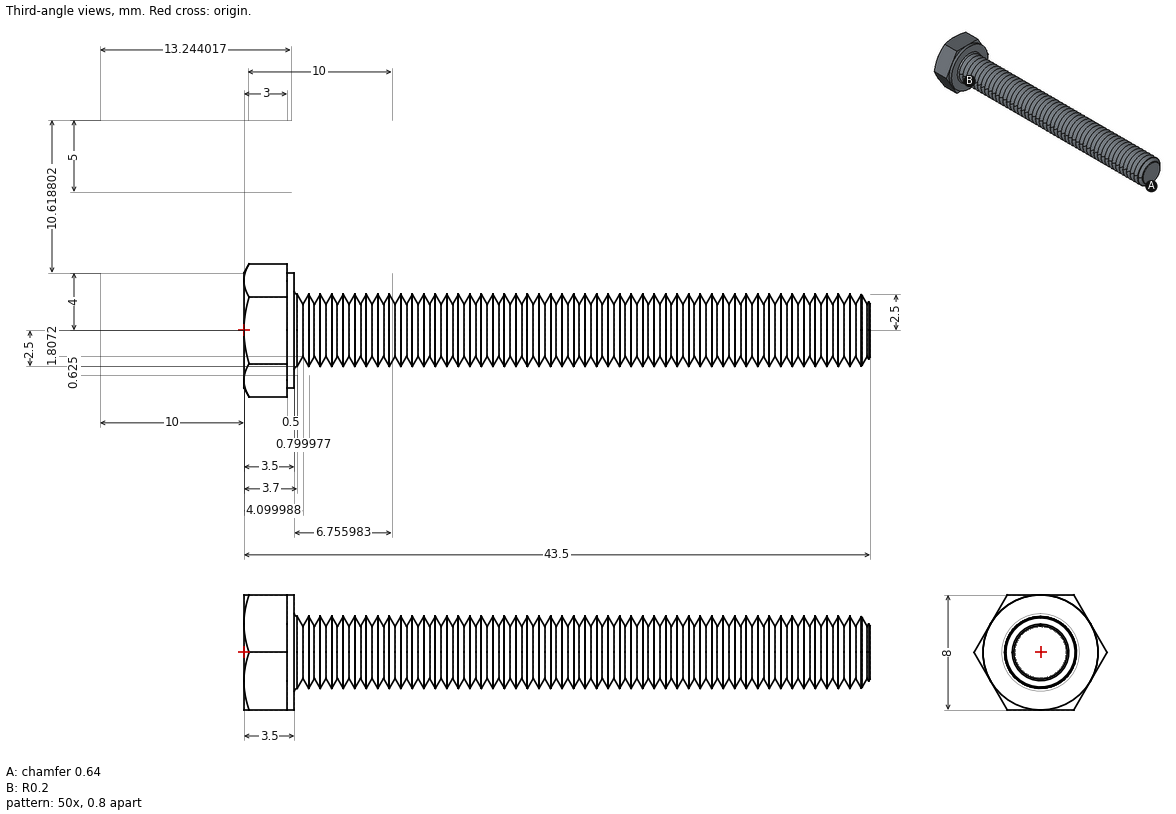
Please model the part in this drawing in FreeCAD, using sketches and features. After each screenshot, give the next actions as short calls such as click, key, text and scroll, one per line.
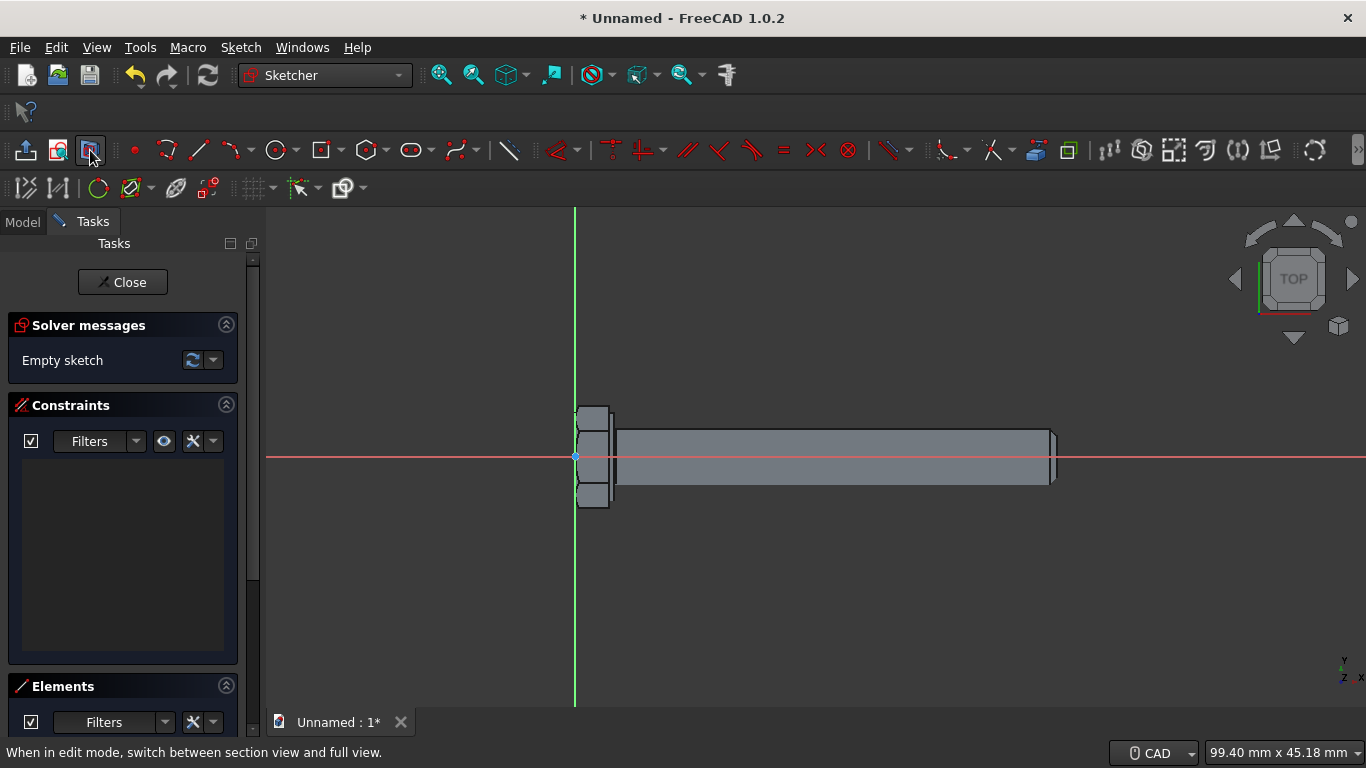
scroll(614, 486, up, 15)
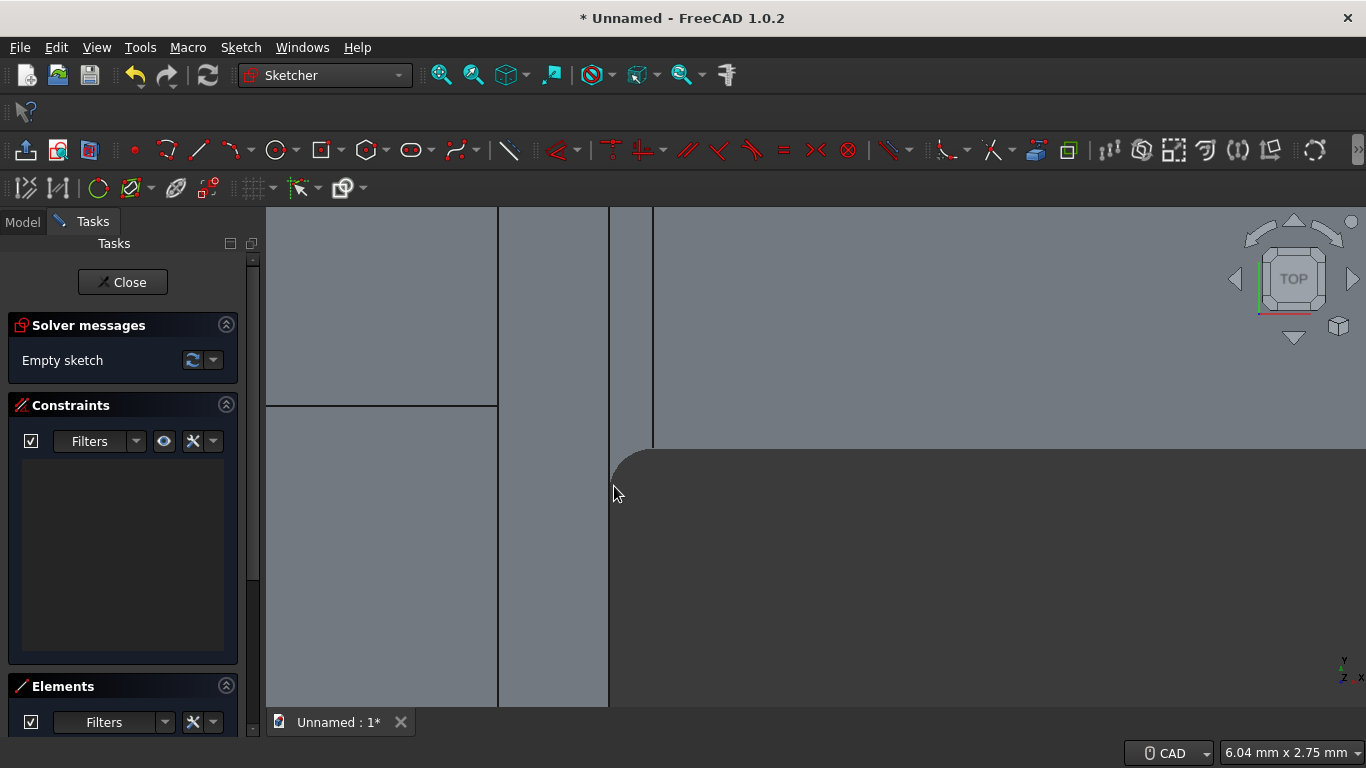
click(168, 150)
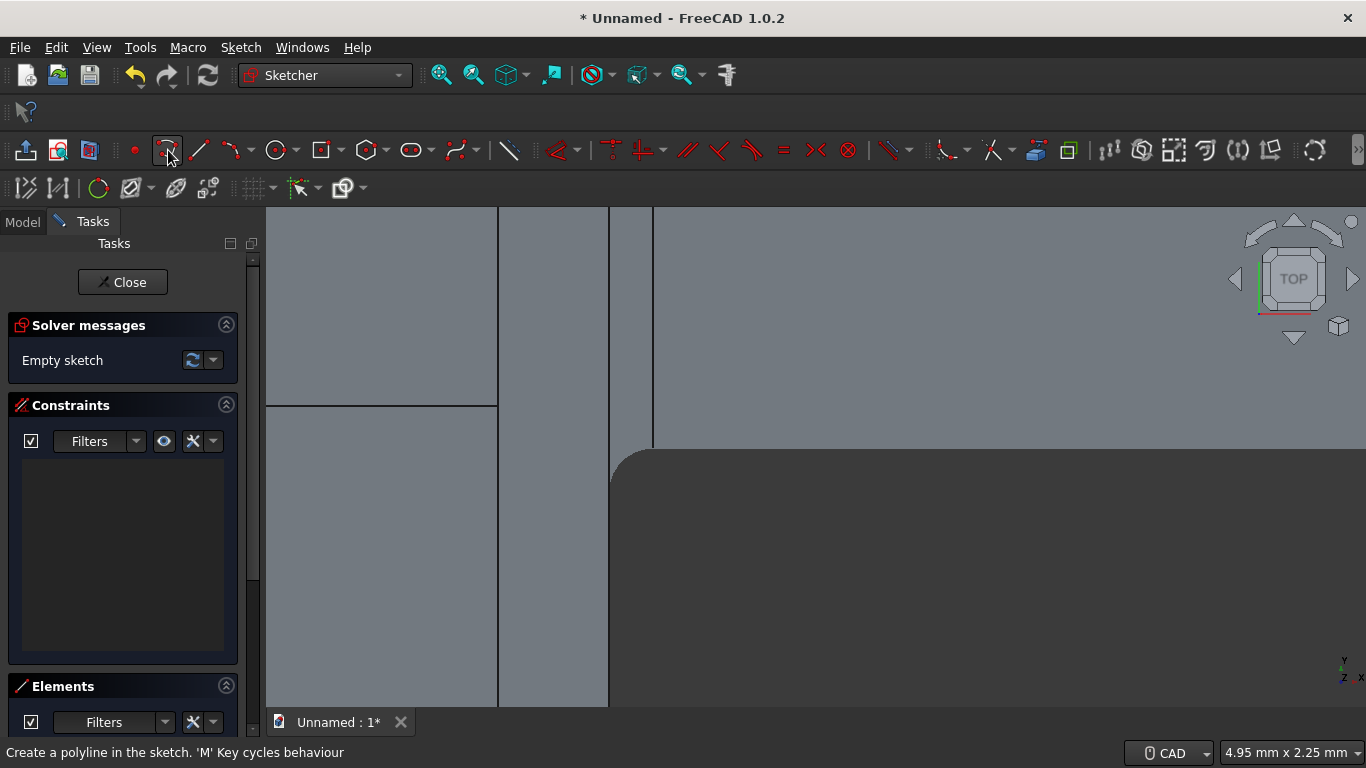
click(653, 449)
click(653, 587)
click(831, 587)
click(831, 449)
click(742, 295)
click(653, 450)
key(Escape)
key(Escape)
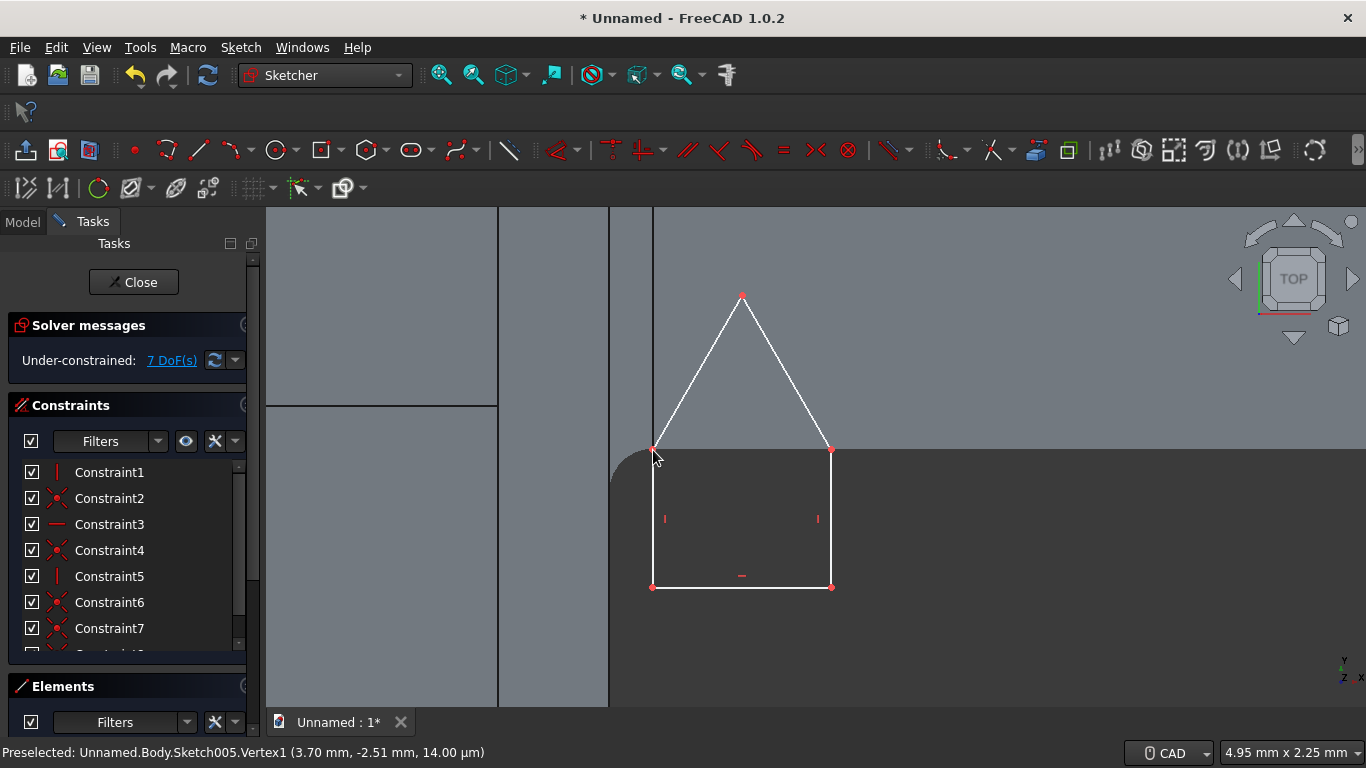
click(556, 150)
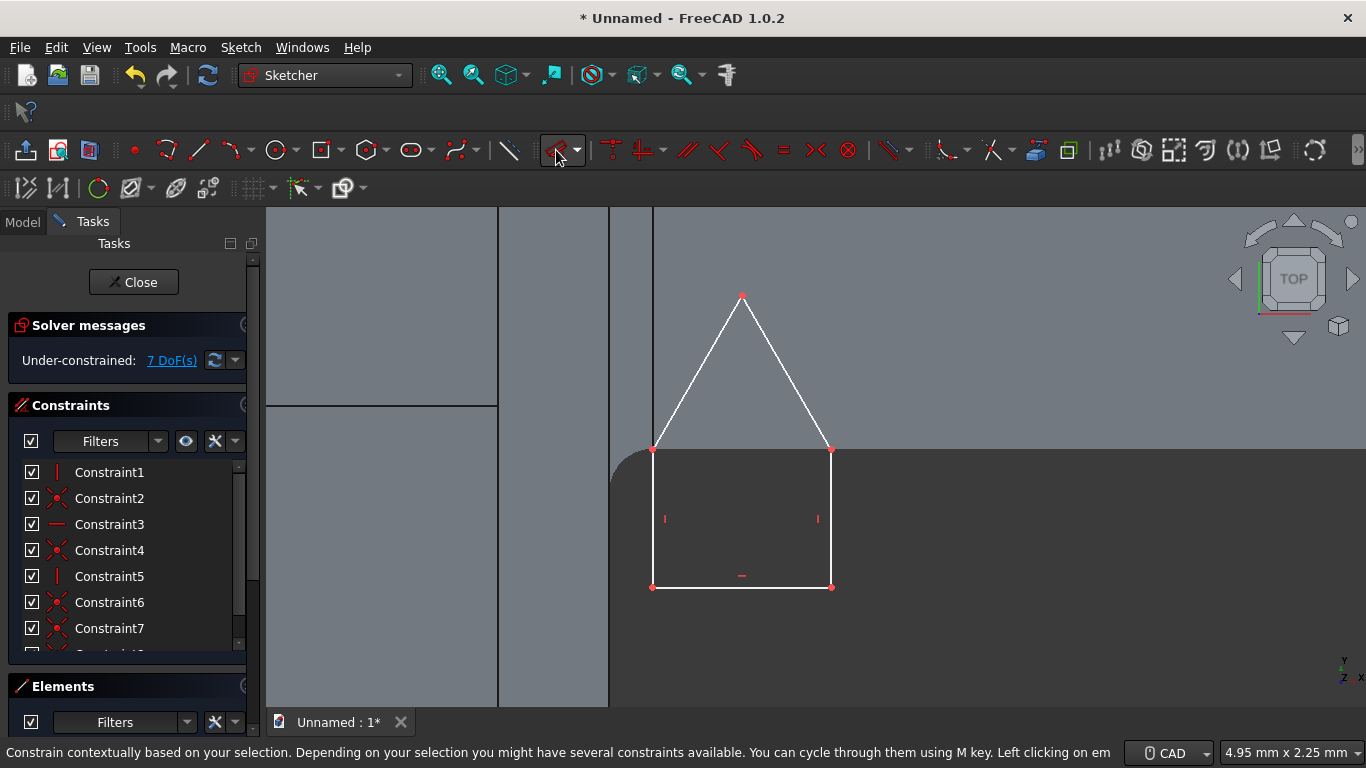
click(653, 450)
click(473, 484)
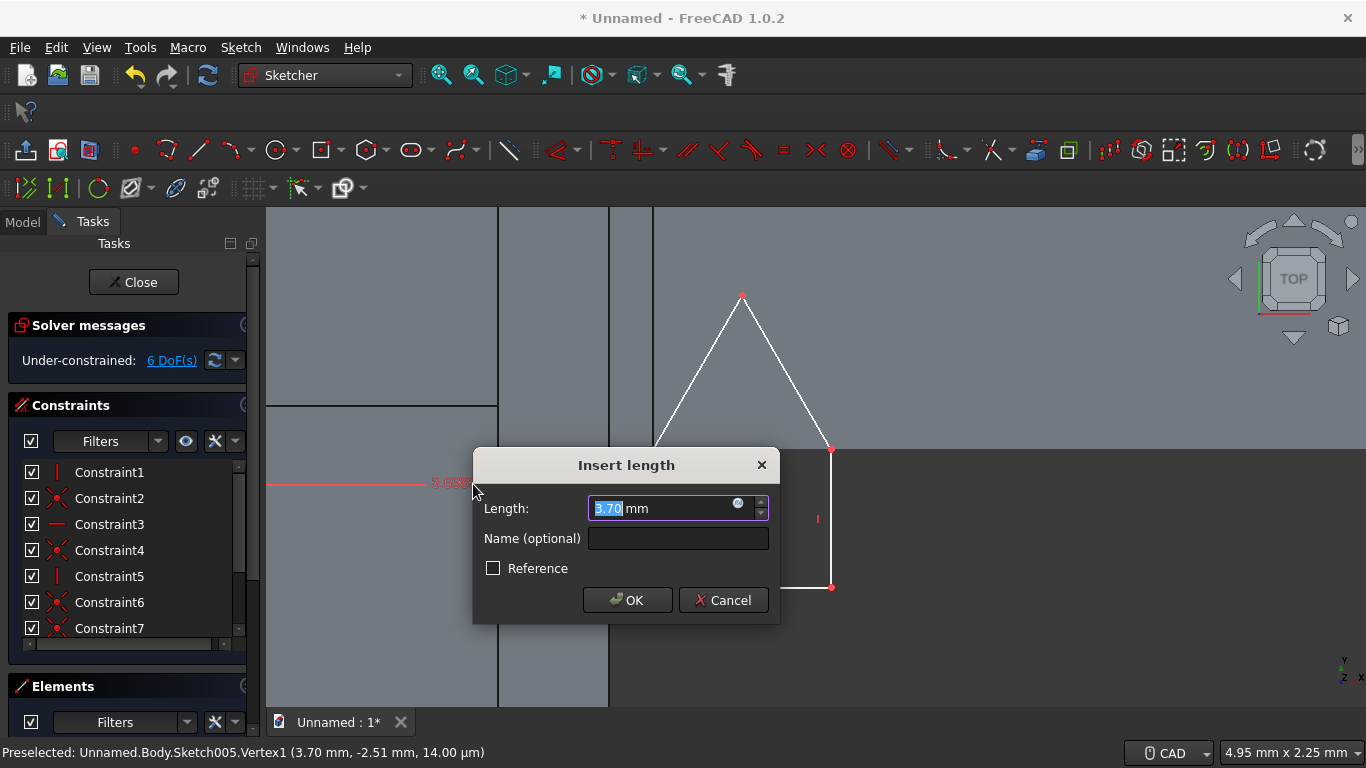
text(3.7)
key(Return)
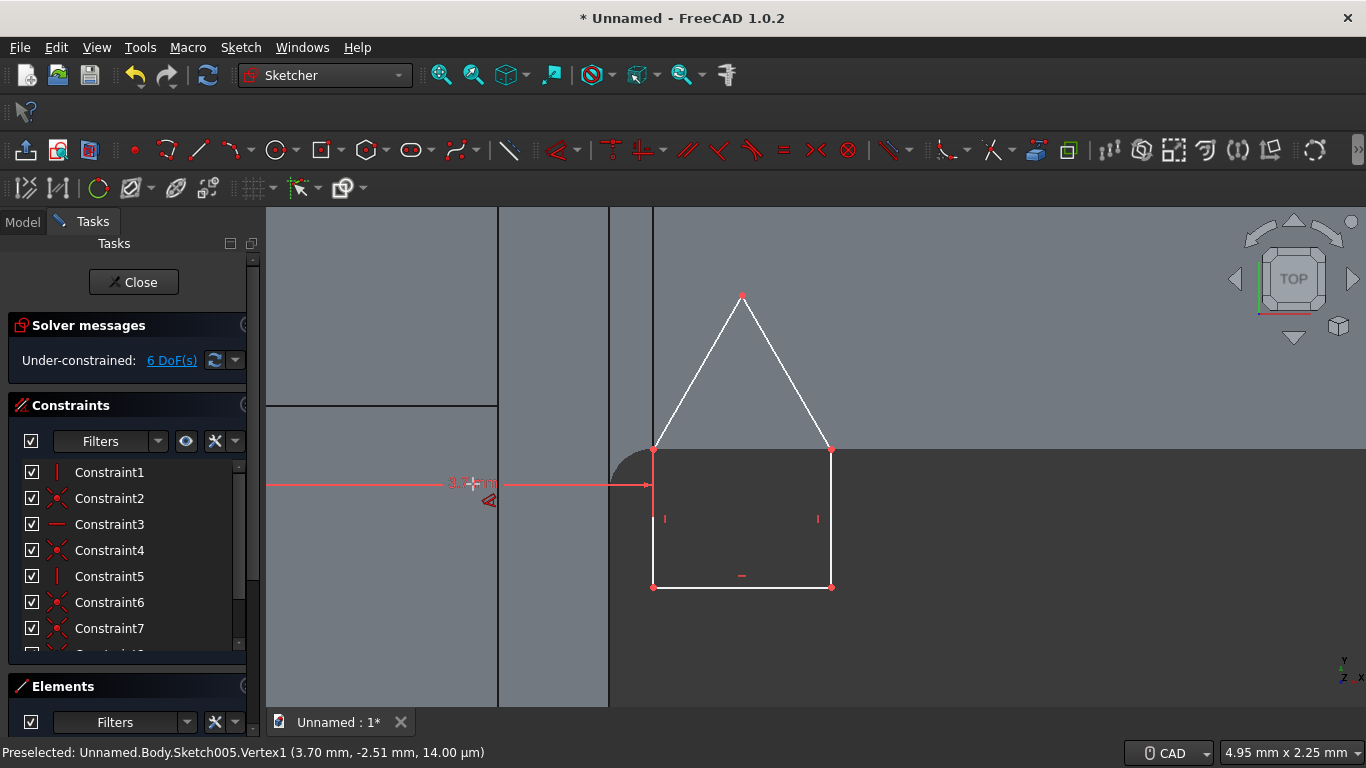
click(653, 450)
click(687, 342)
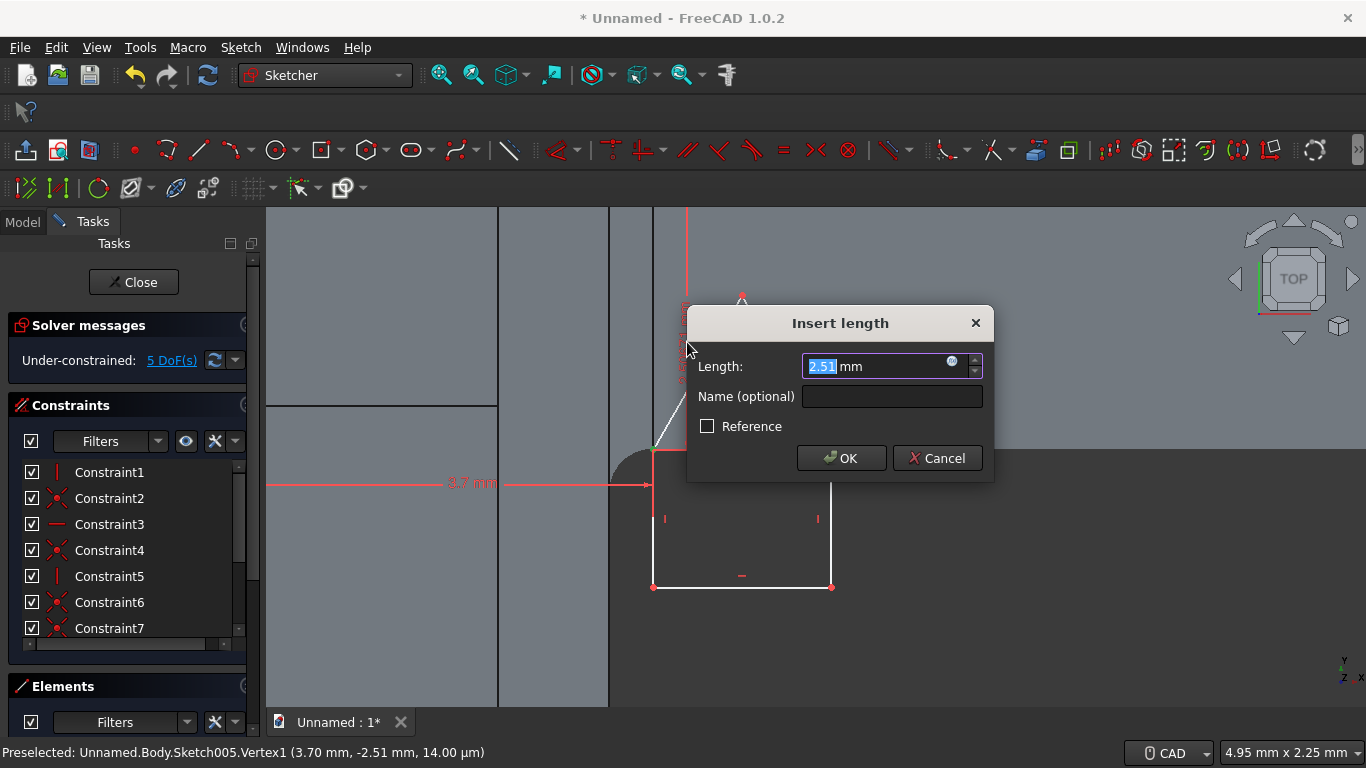
text(2.5)
key(Return)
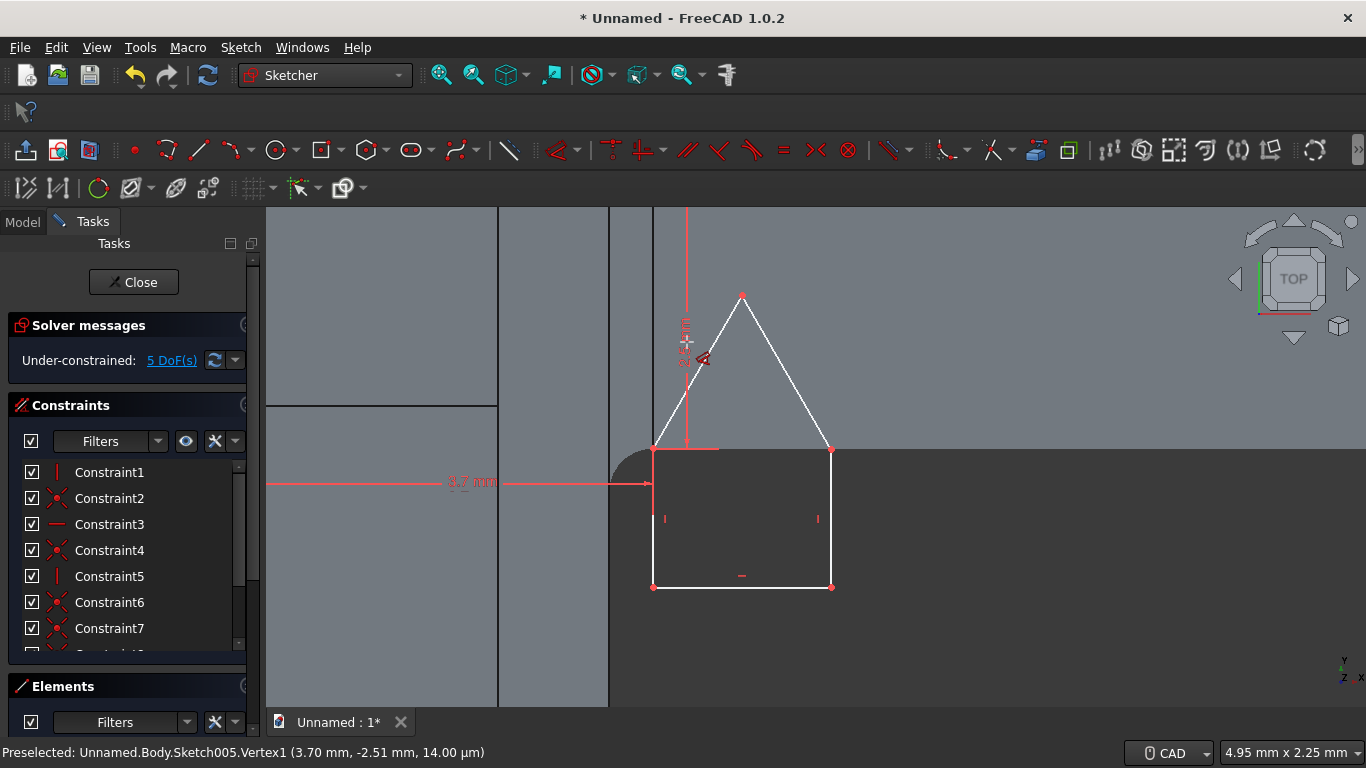
click(831, 450)
click(865, 342)